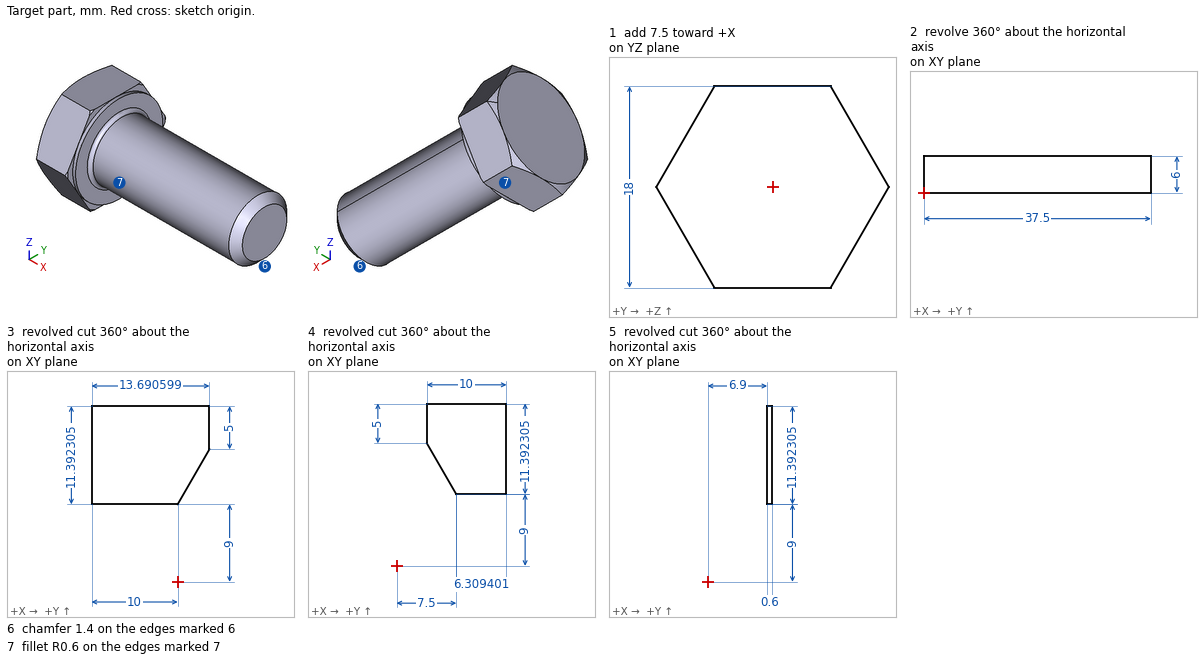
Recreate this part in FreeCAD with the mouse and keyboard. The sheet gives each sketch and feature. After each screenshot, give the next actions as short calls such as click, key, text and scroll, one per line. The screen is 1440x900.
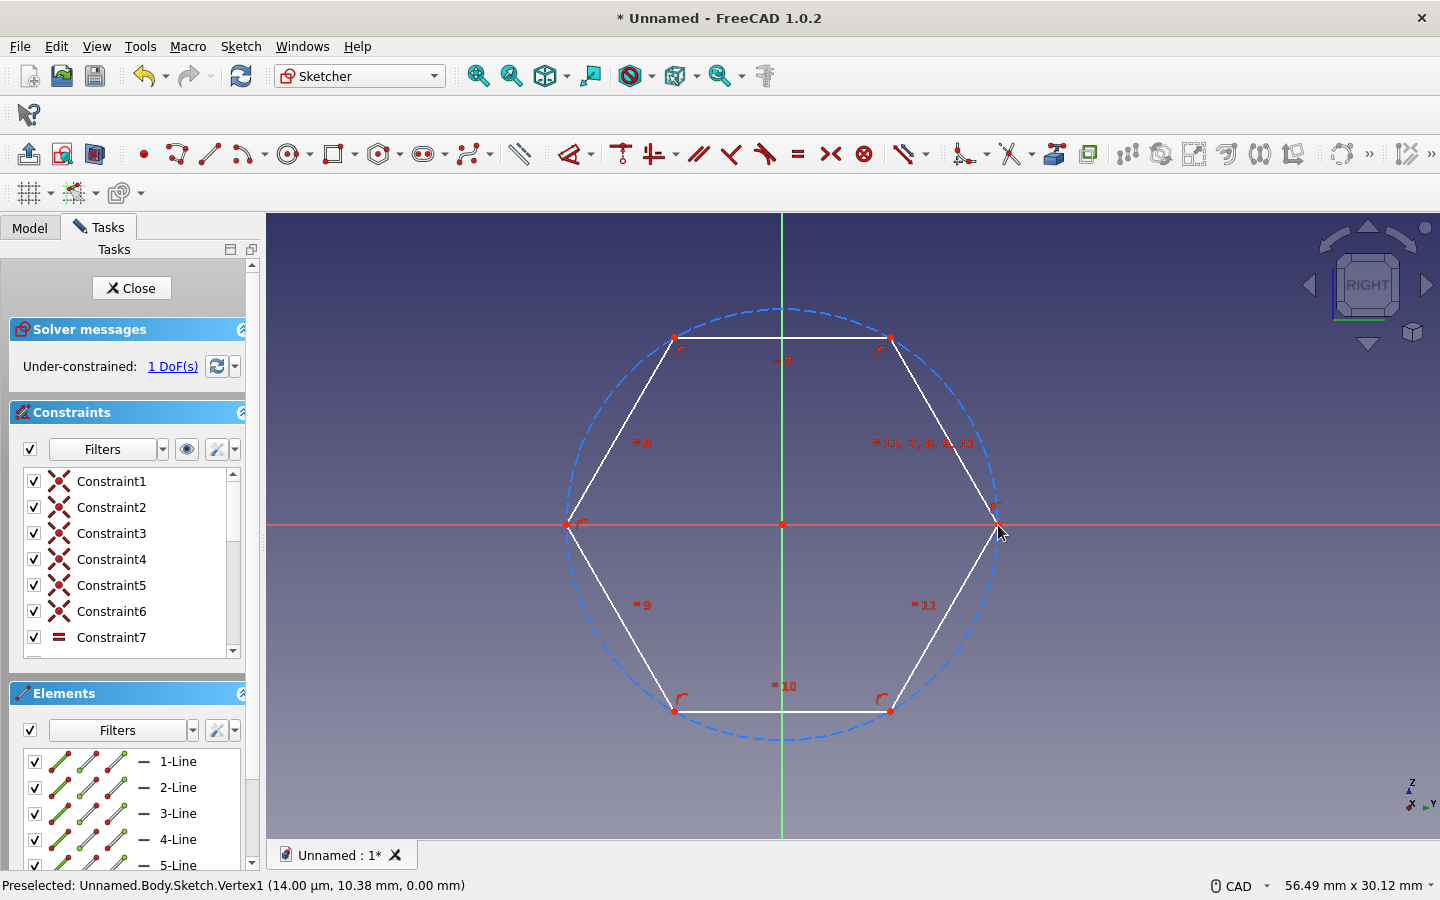
click(568, 154)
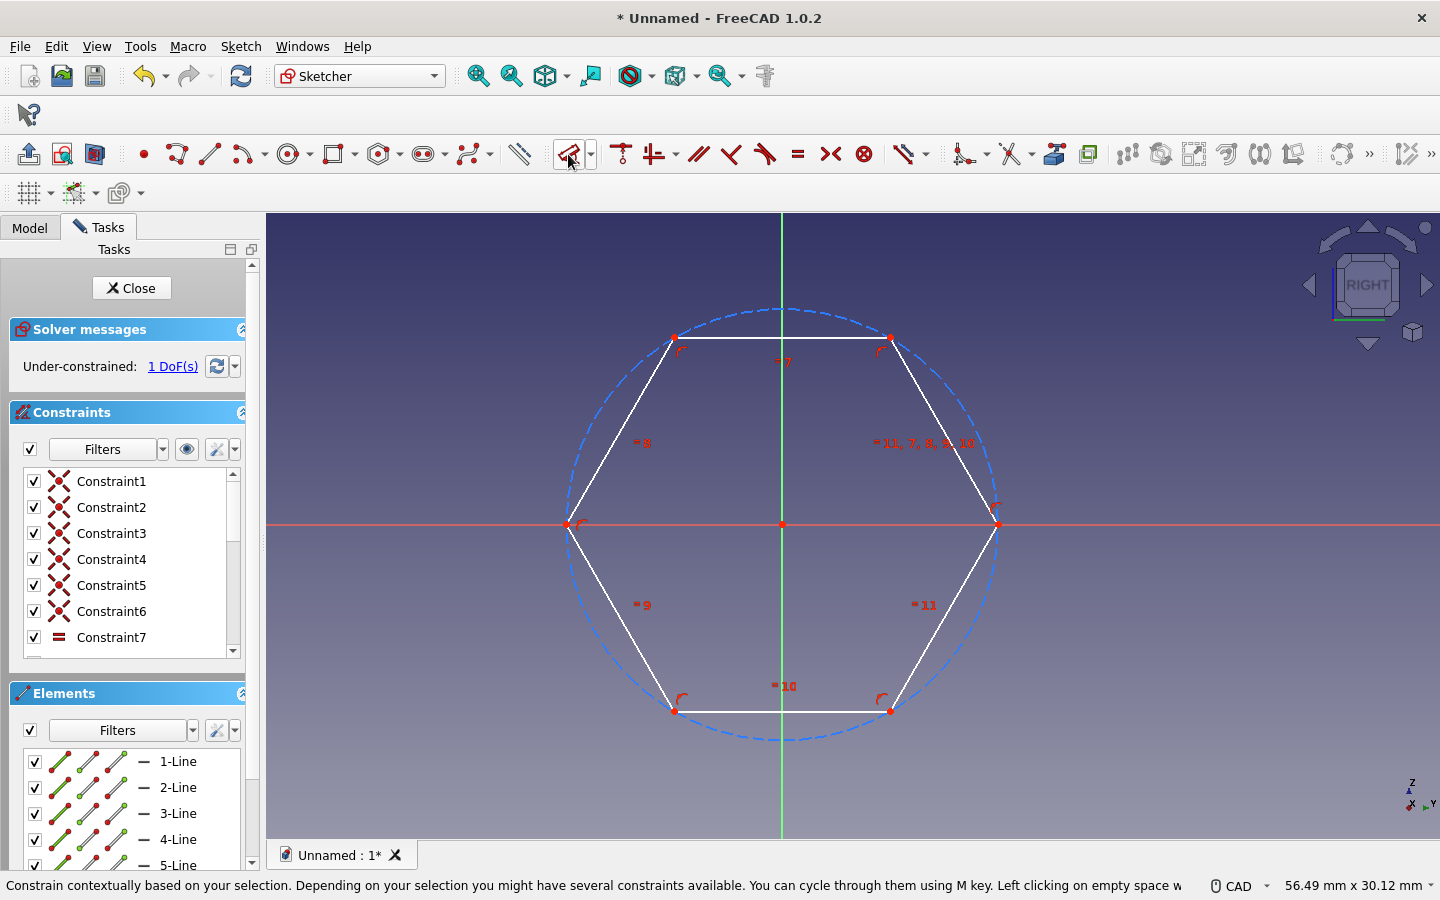
click(674, 712)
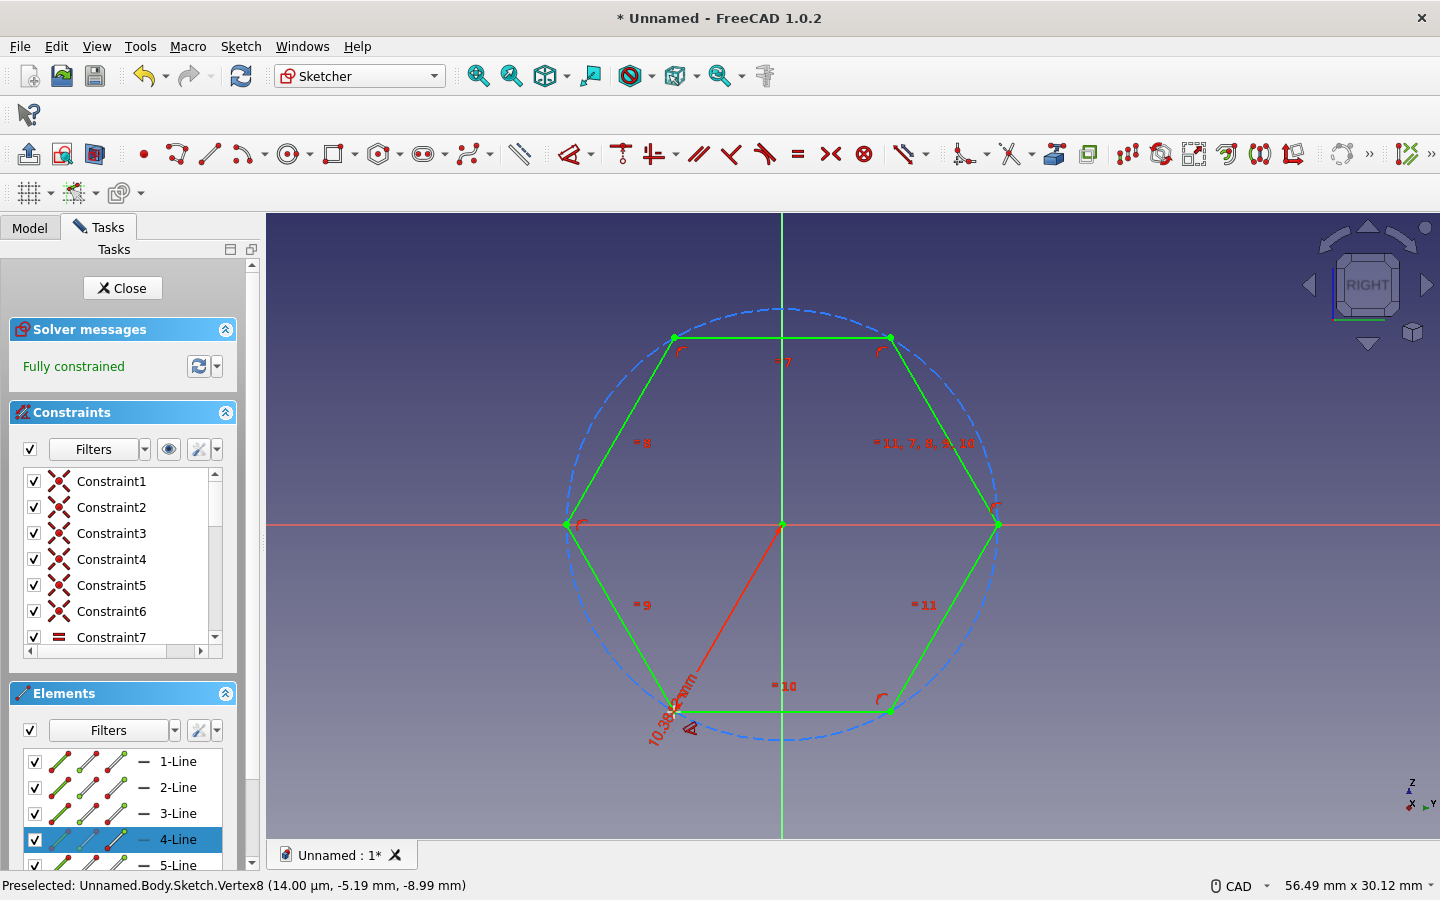
click(890, 338)
click(924, 439)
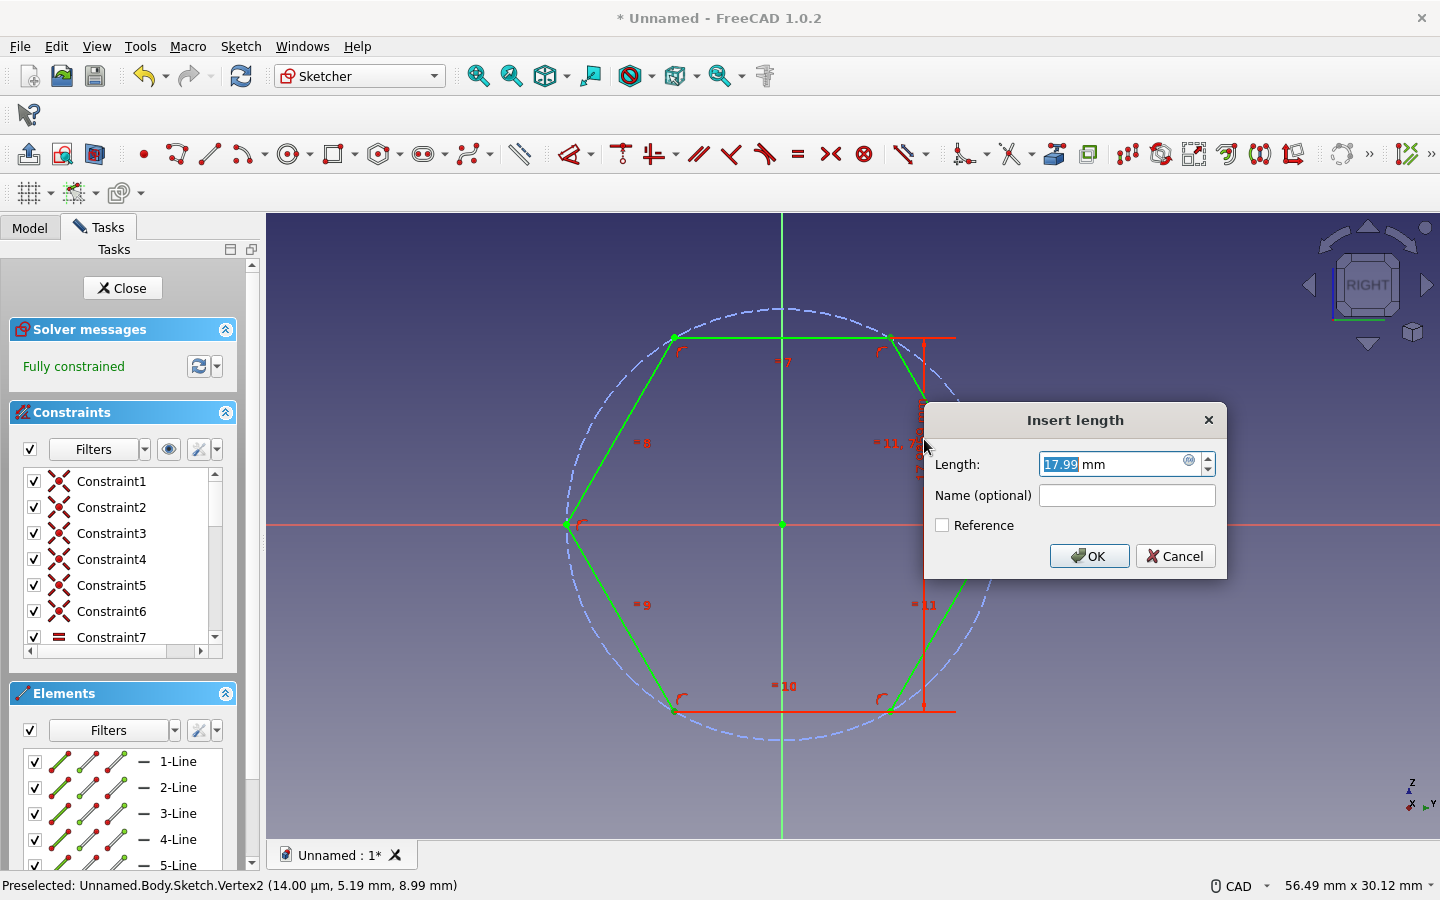
text(18)
key(Return)
key(Escape)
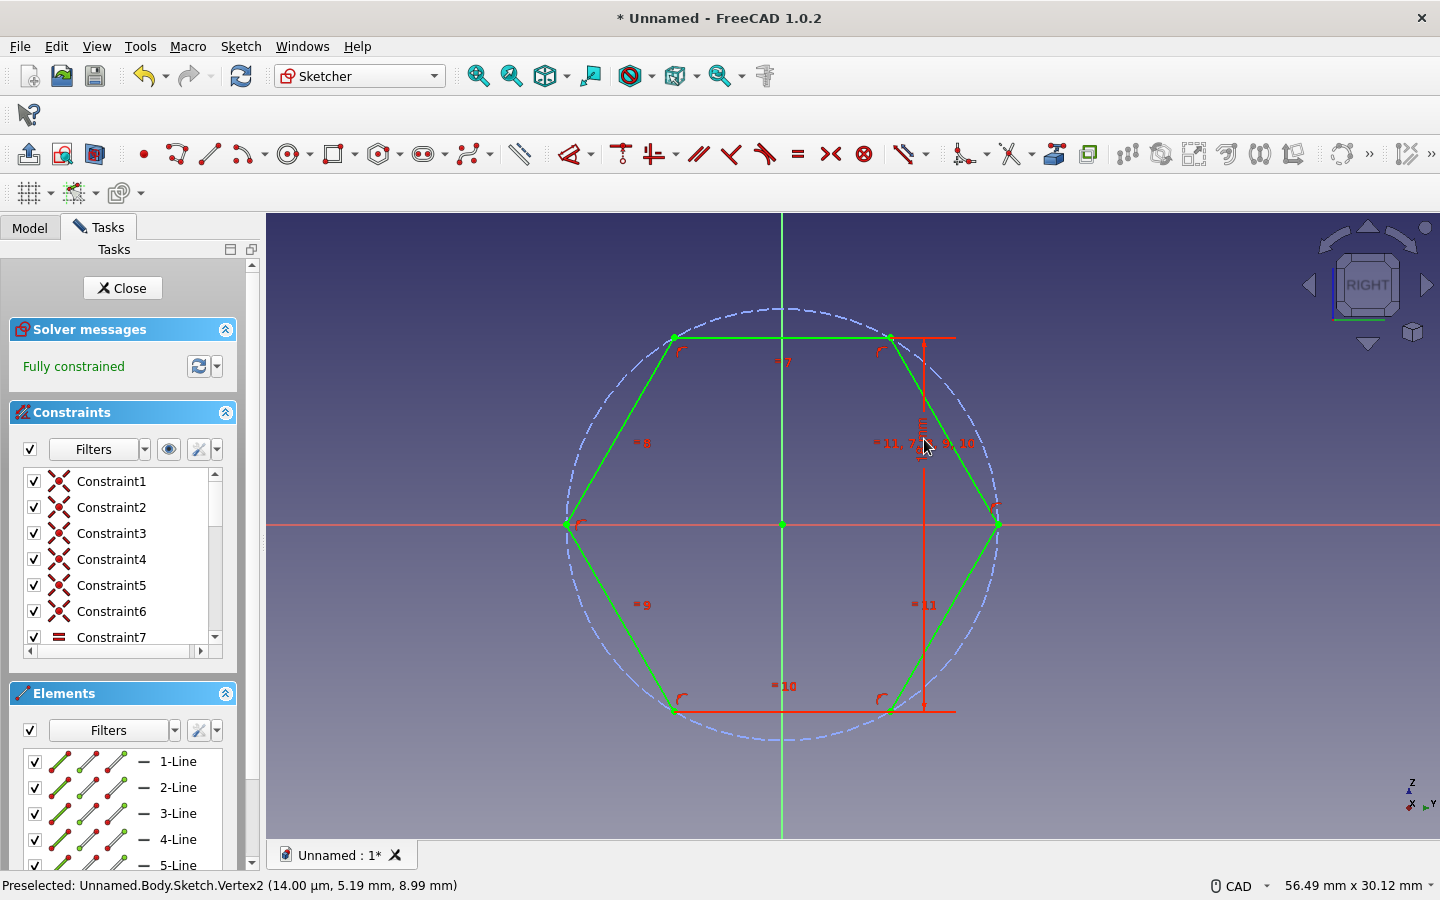
click(123, 288)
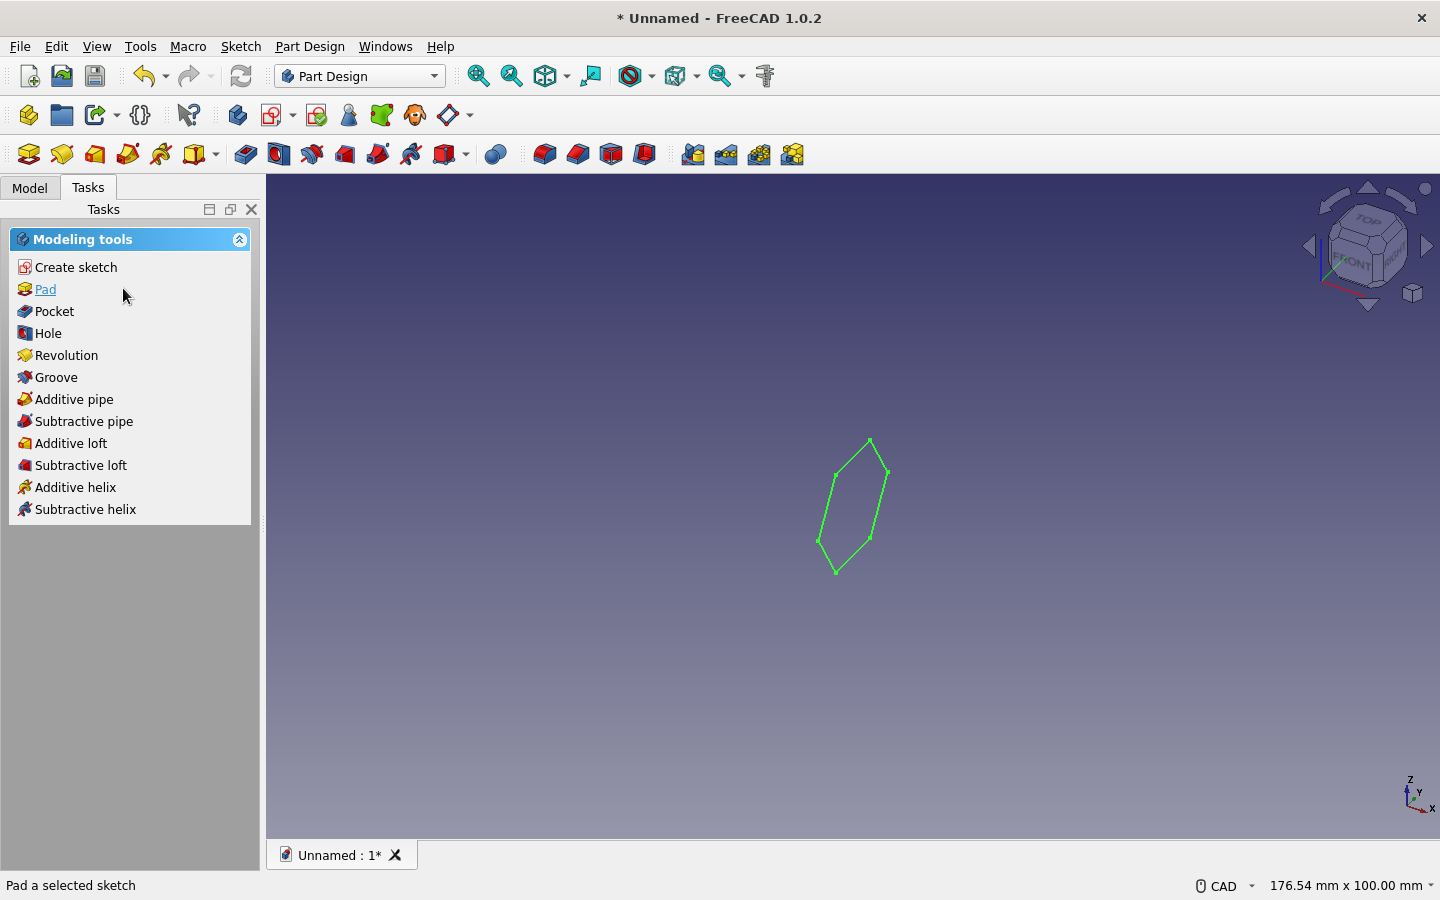
click(29, 154)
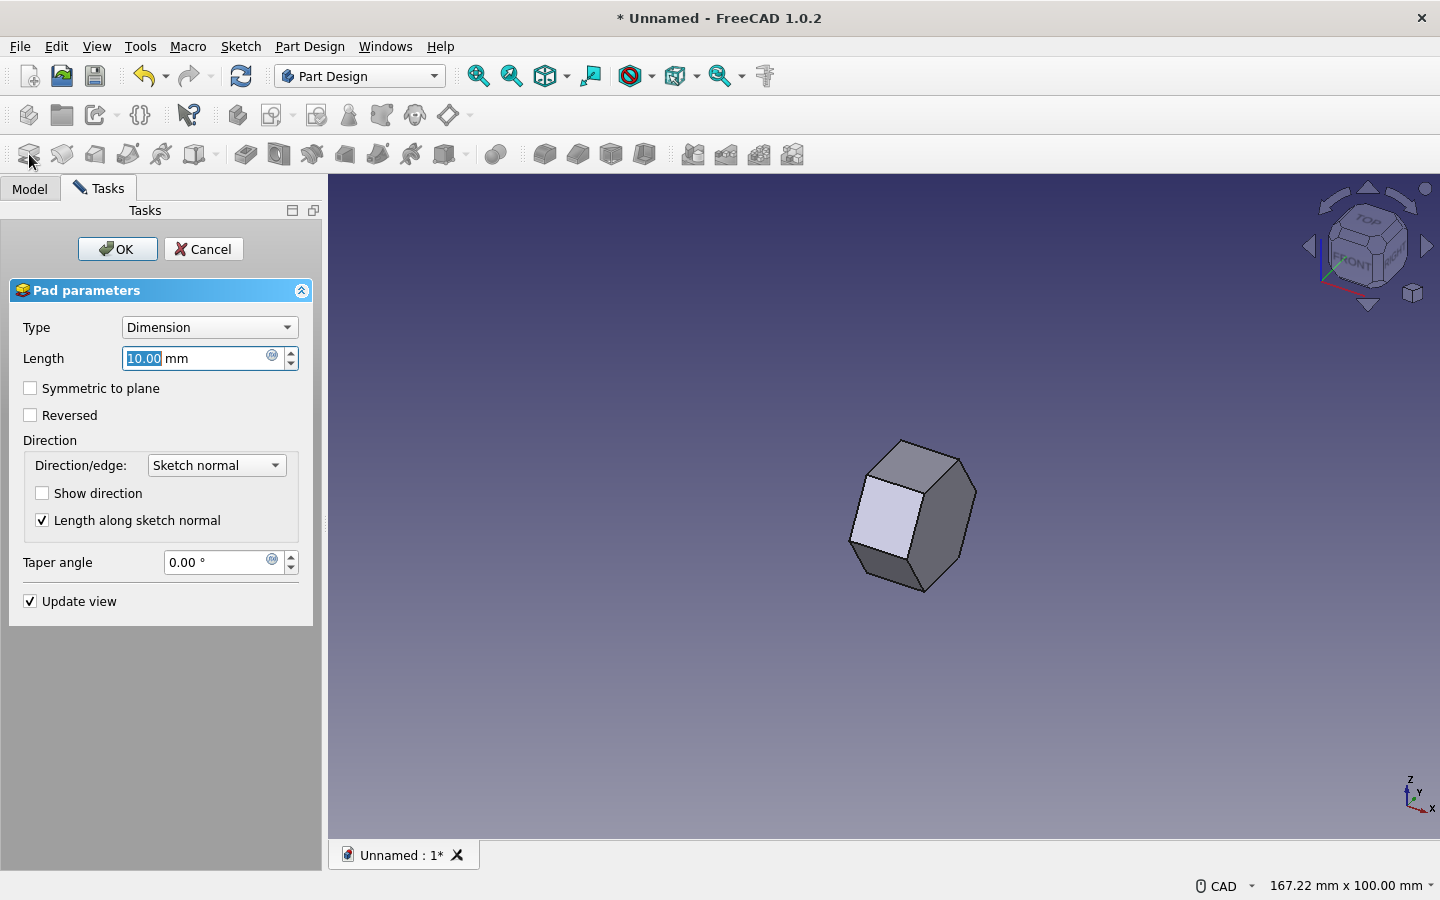
text(7.5)
key(Tab)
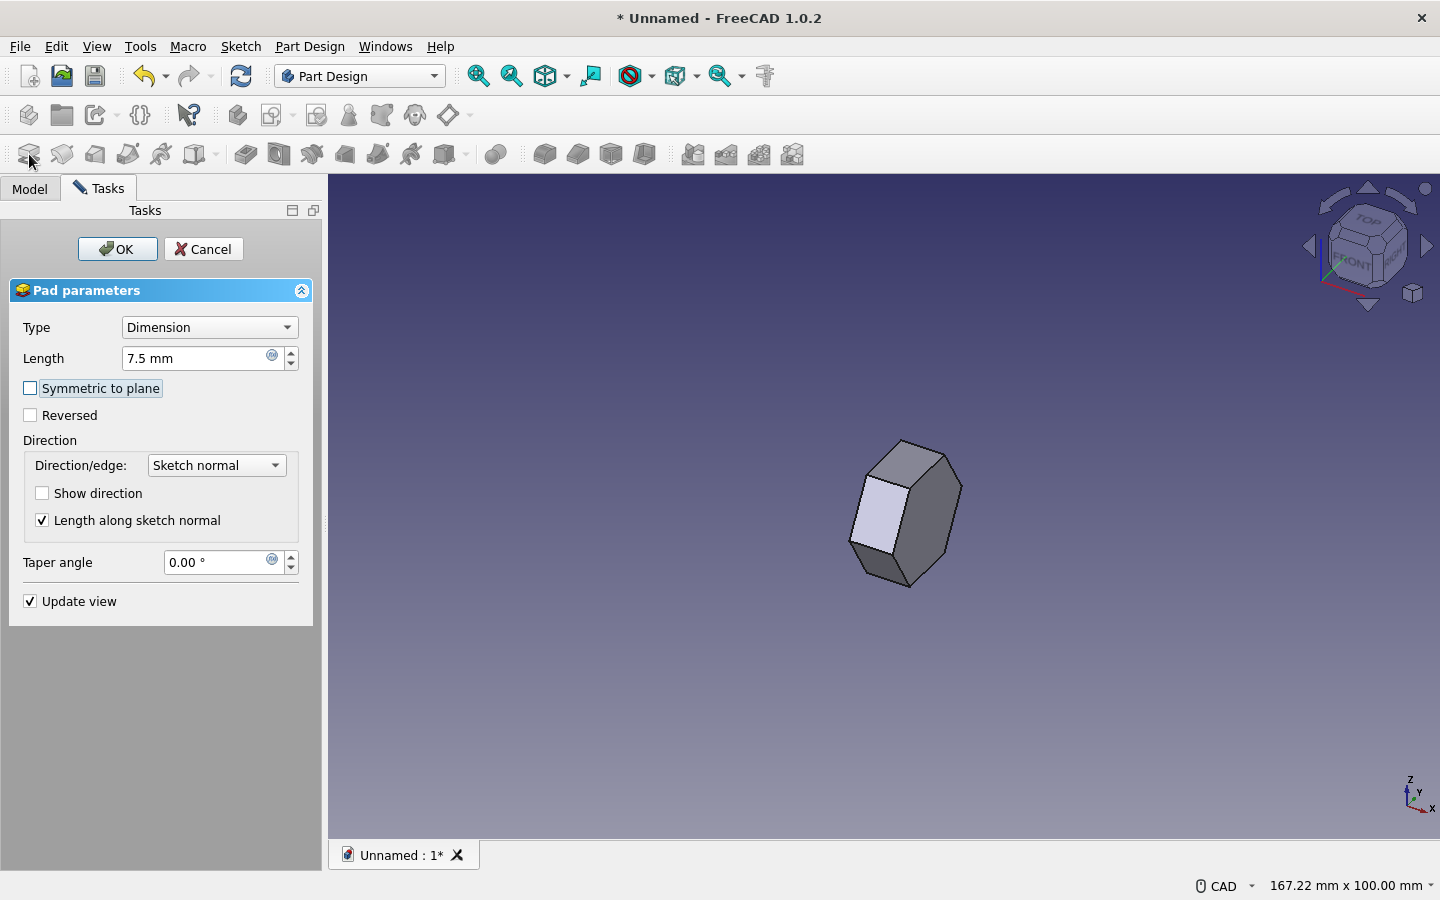
click(118, 249)